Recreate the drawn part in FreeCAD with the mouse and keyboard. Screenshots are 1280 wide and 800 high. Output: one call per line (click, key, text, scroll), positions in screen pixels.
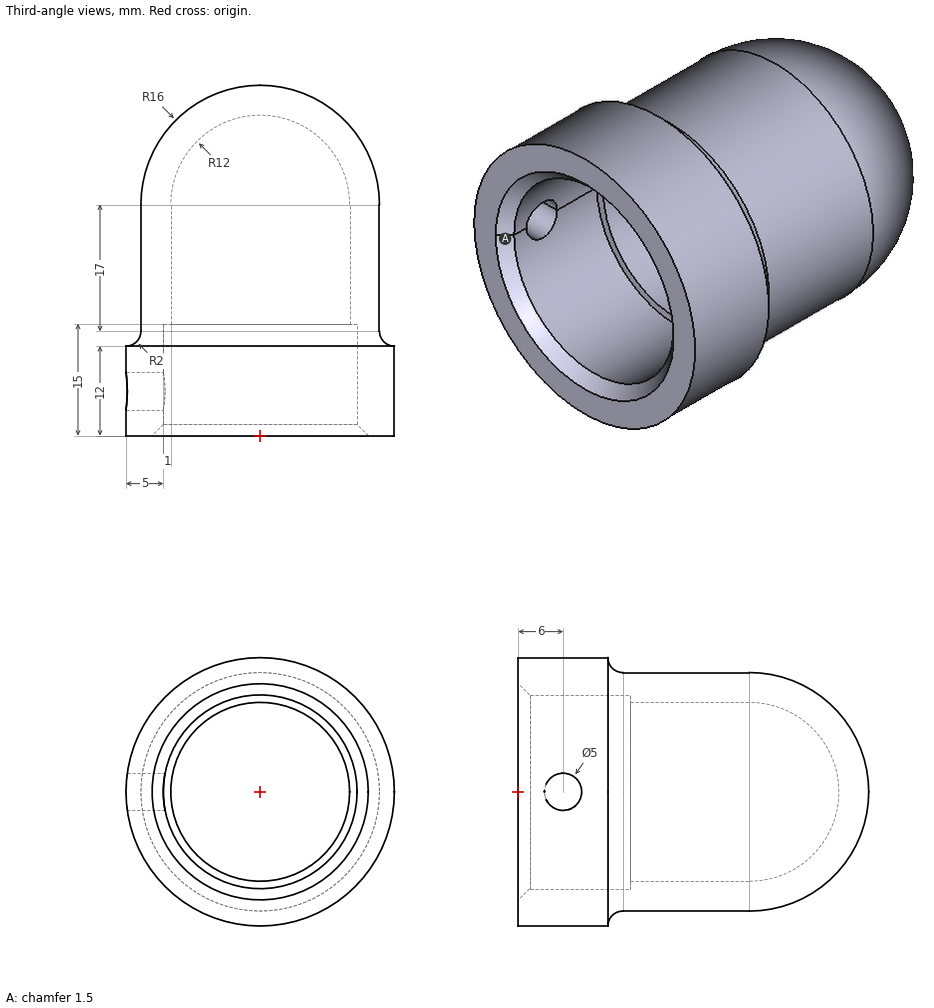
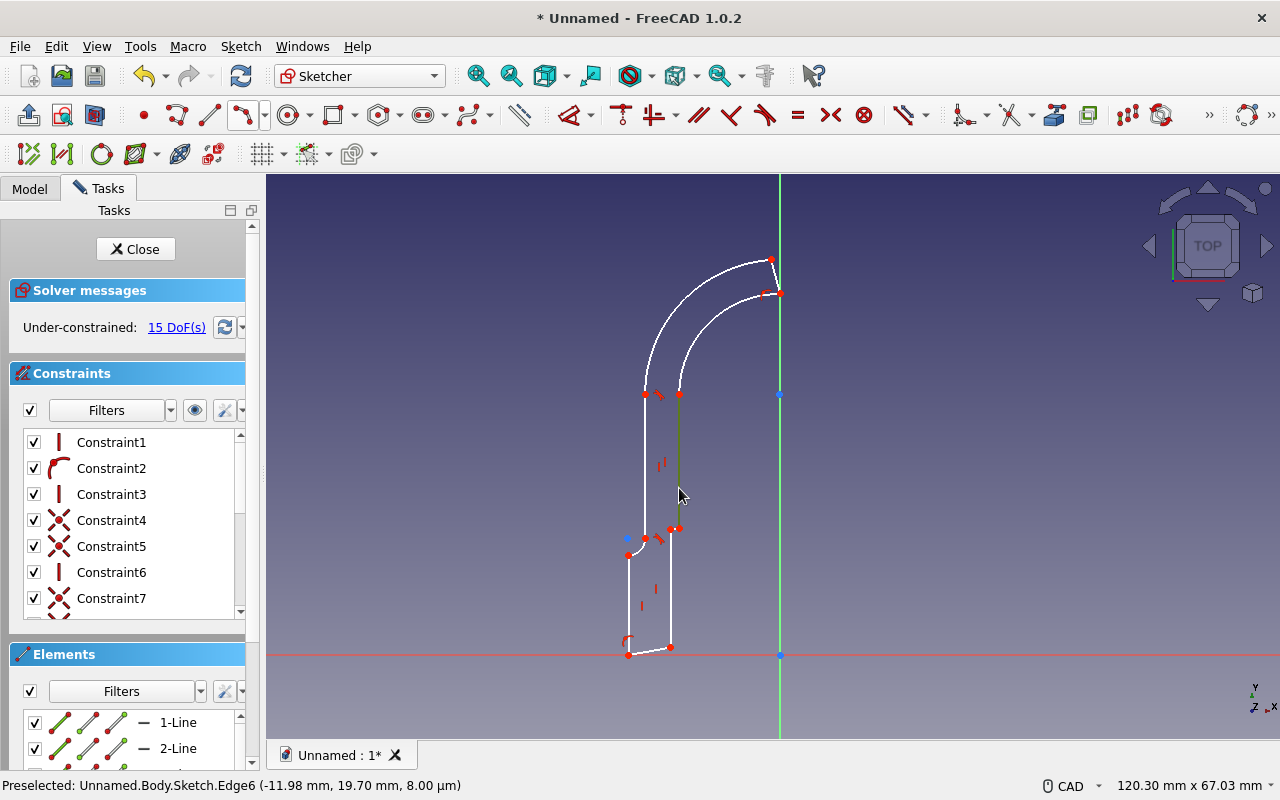
click(735, 305)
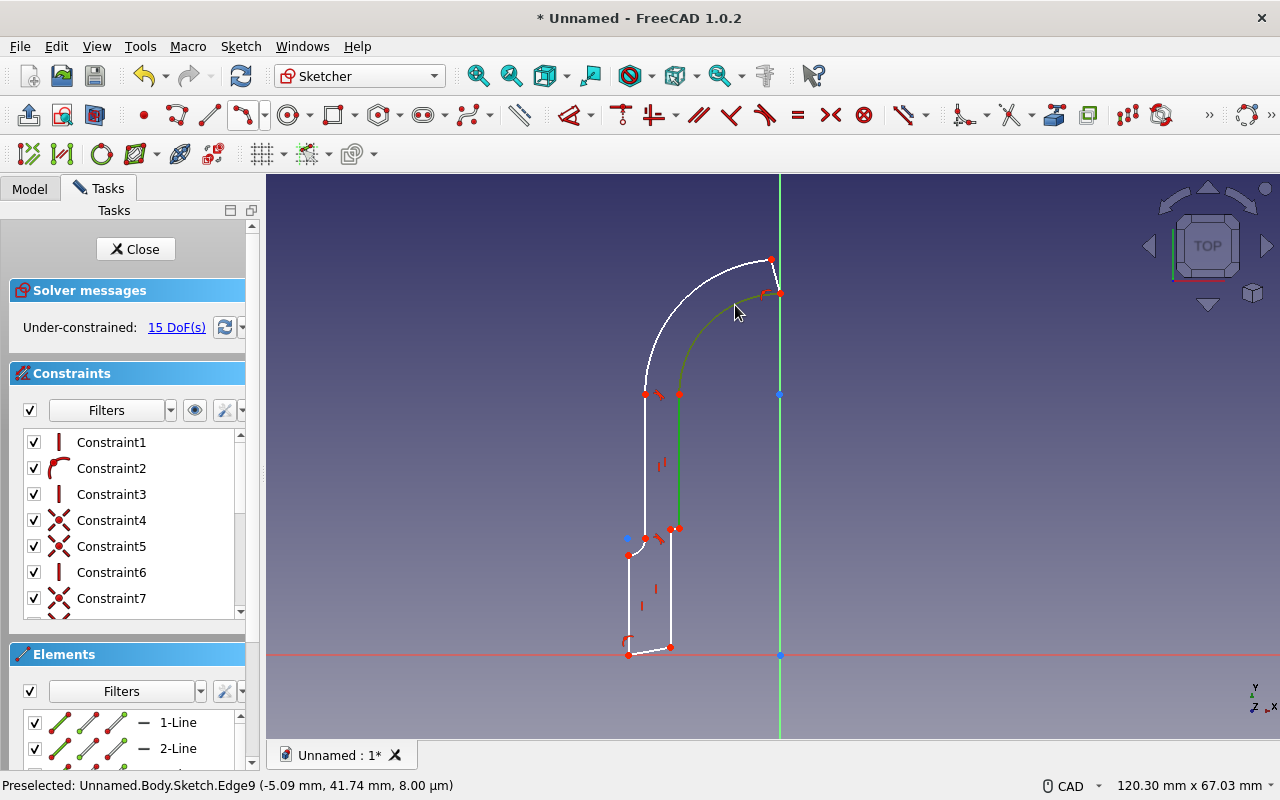
key(t)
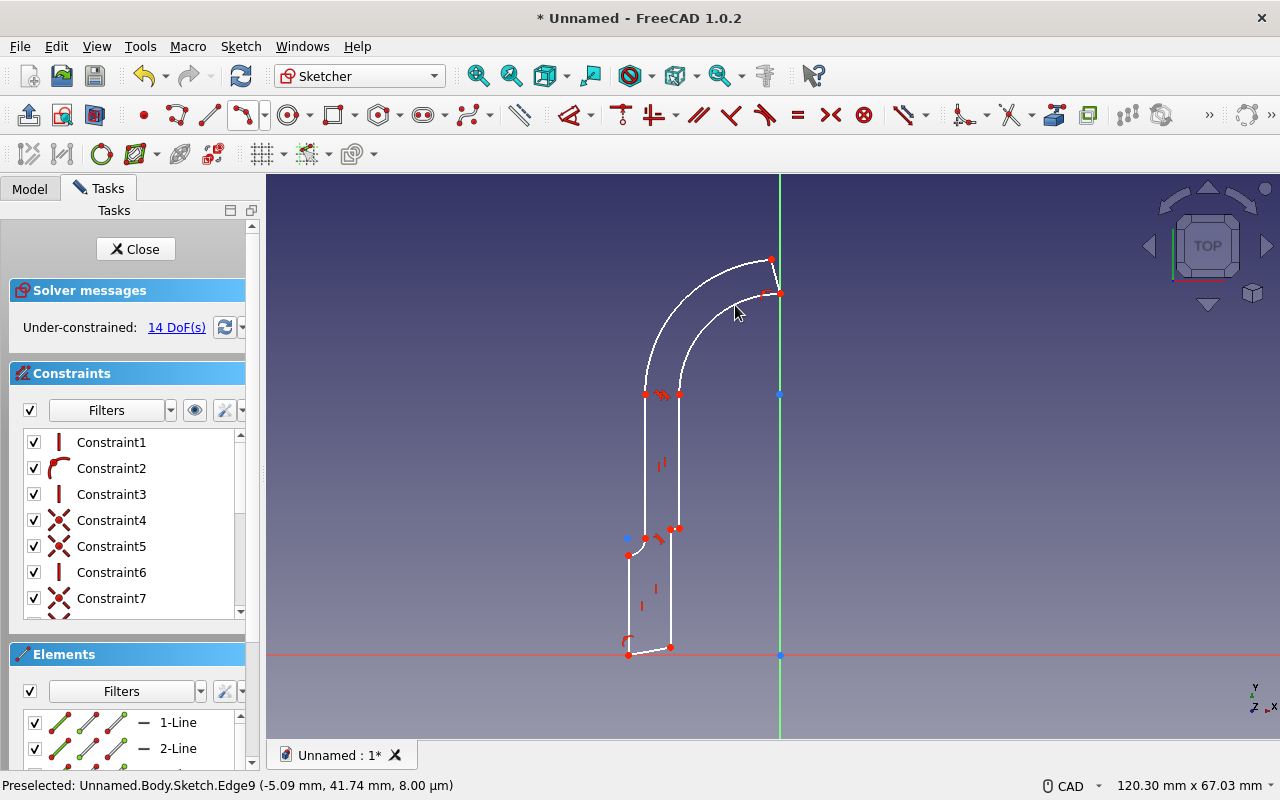
click(641, 653)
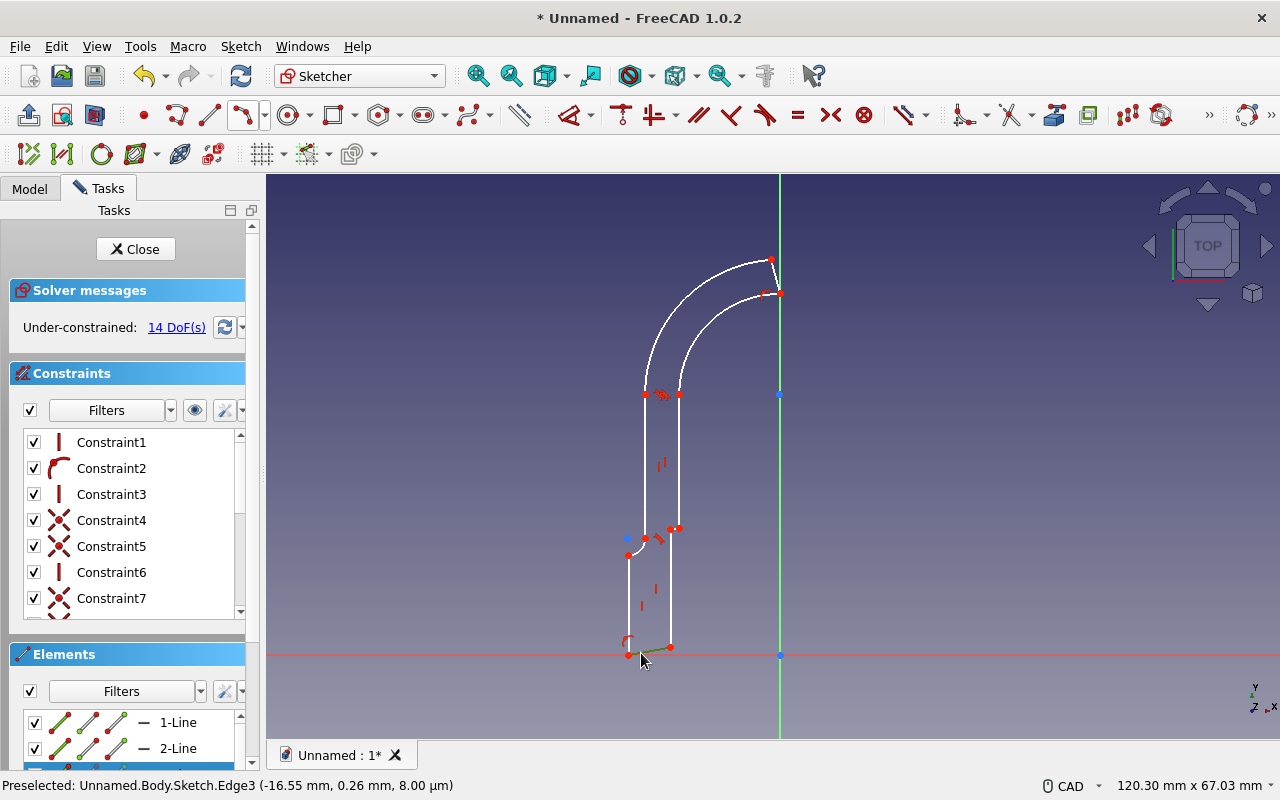
click(676, 116)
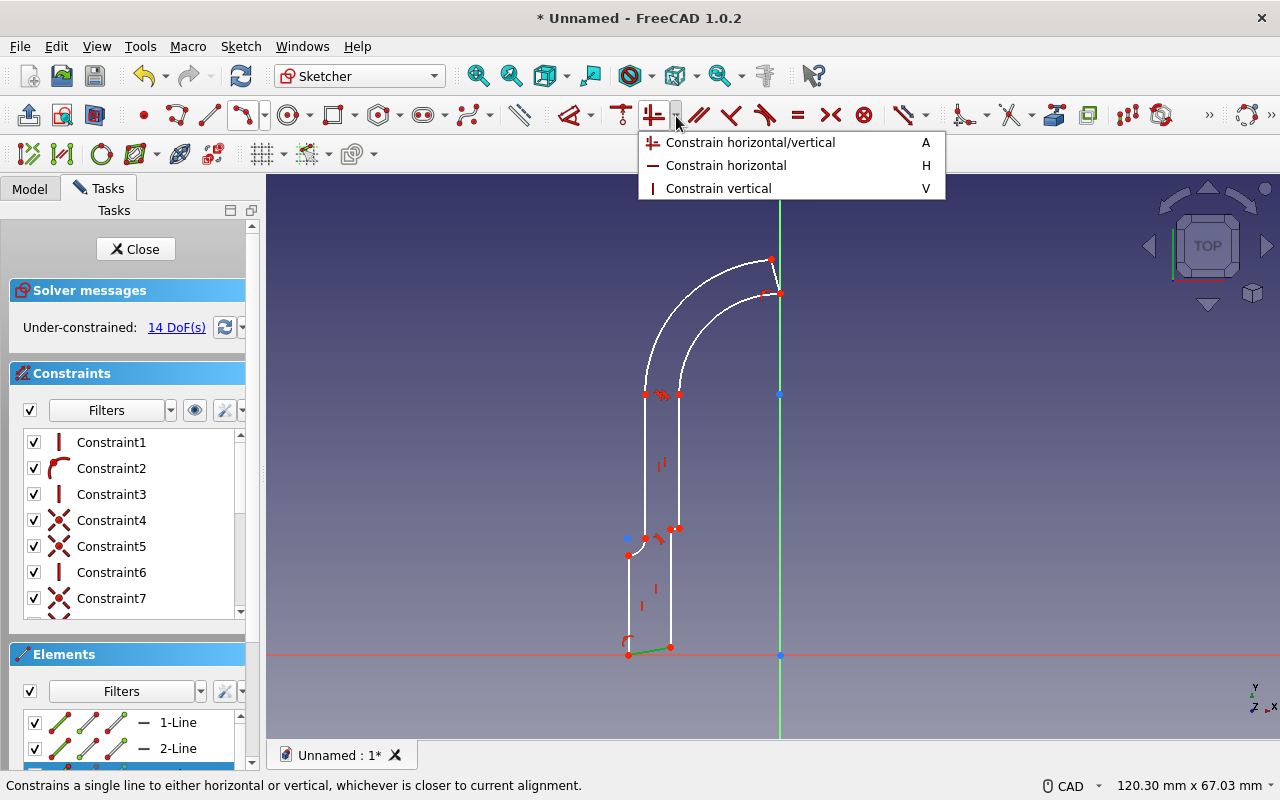
click(792, 166)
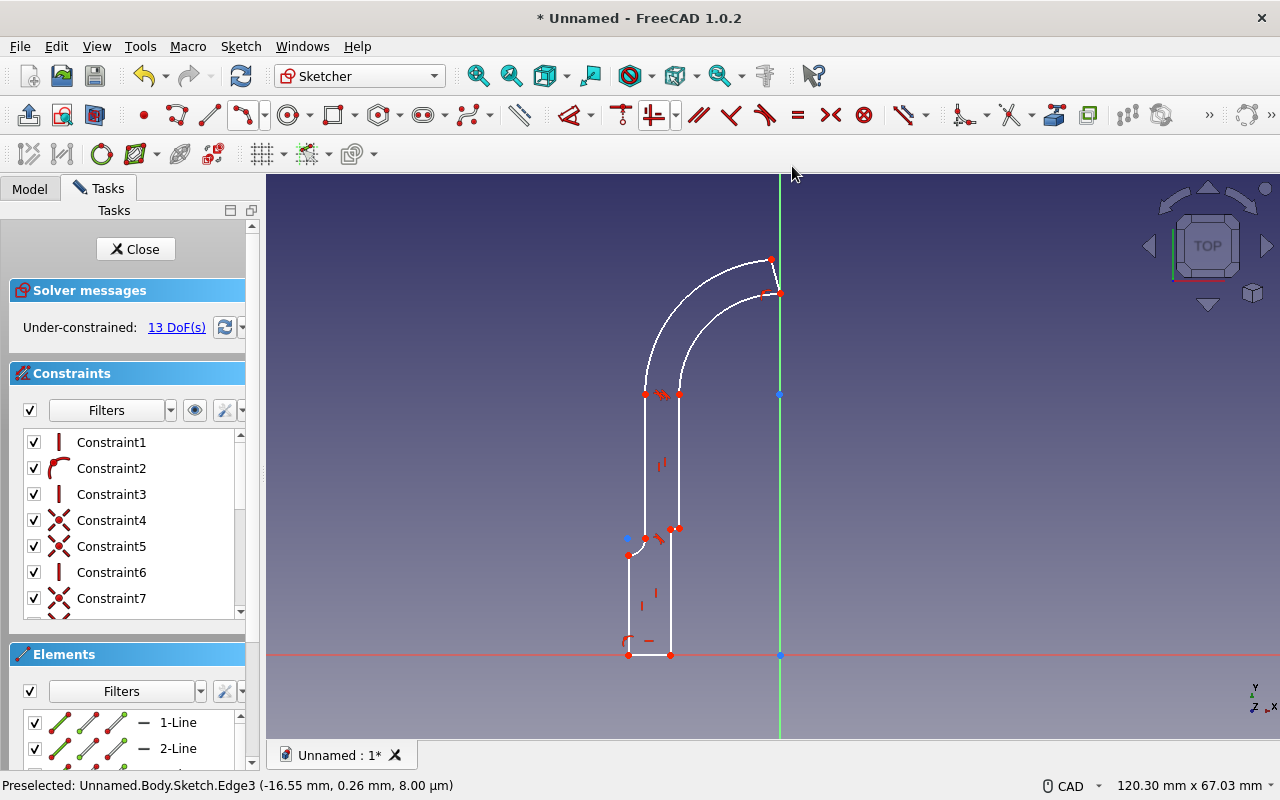
scroll(675, 529, up, 6)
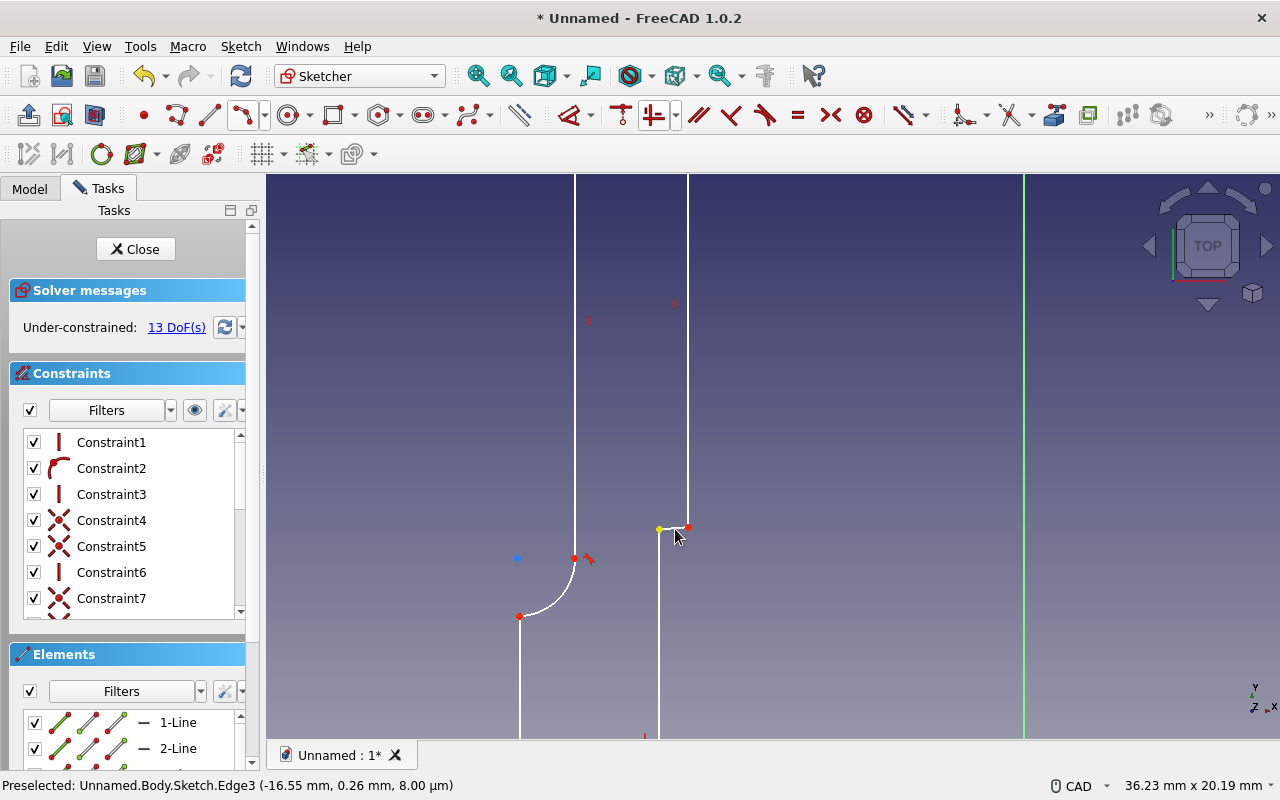
click(674, 528)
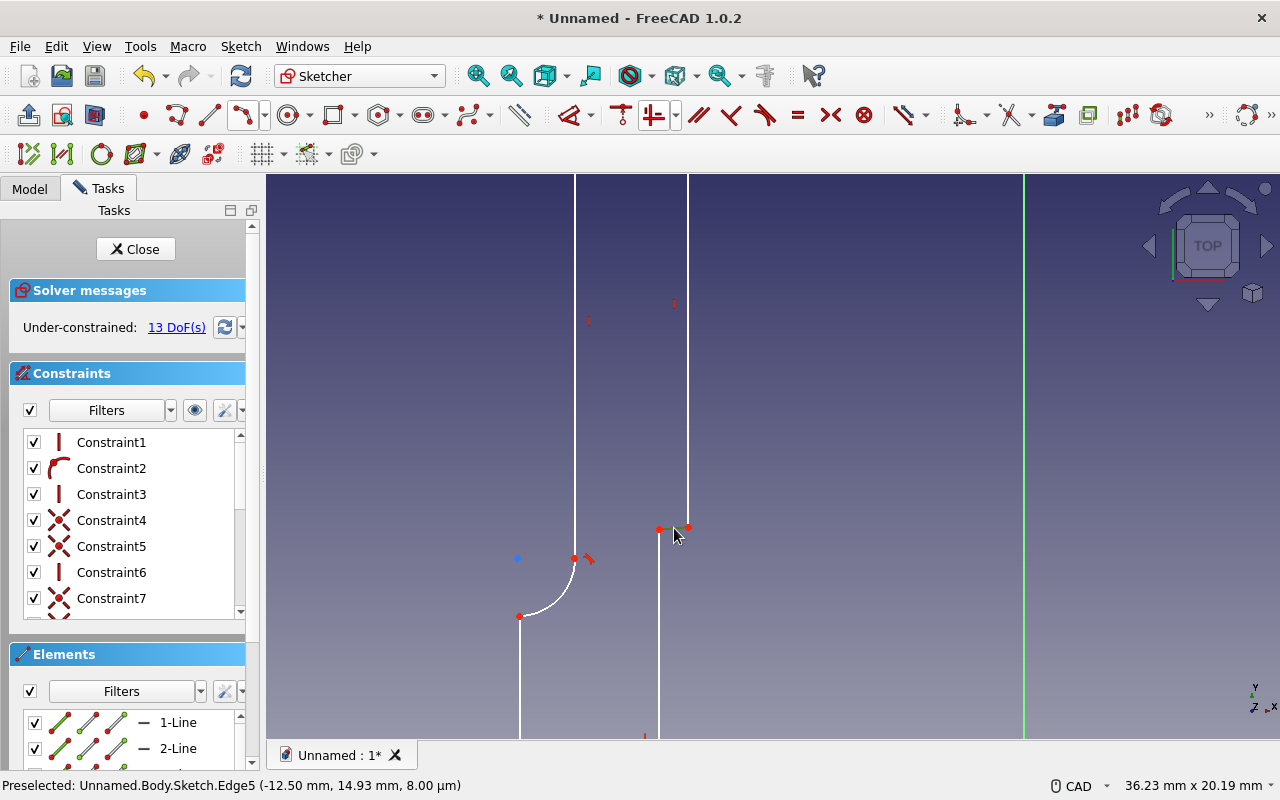
key(h)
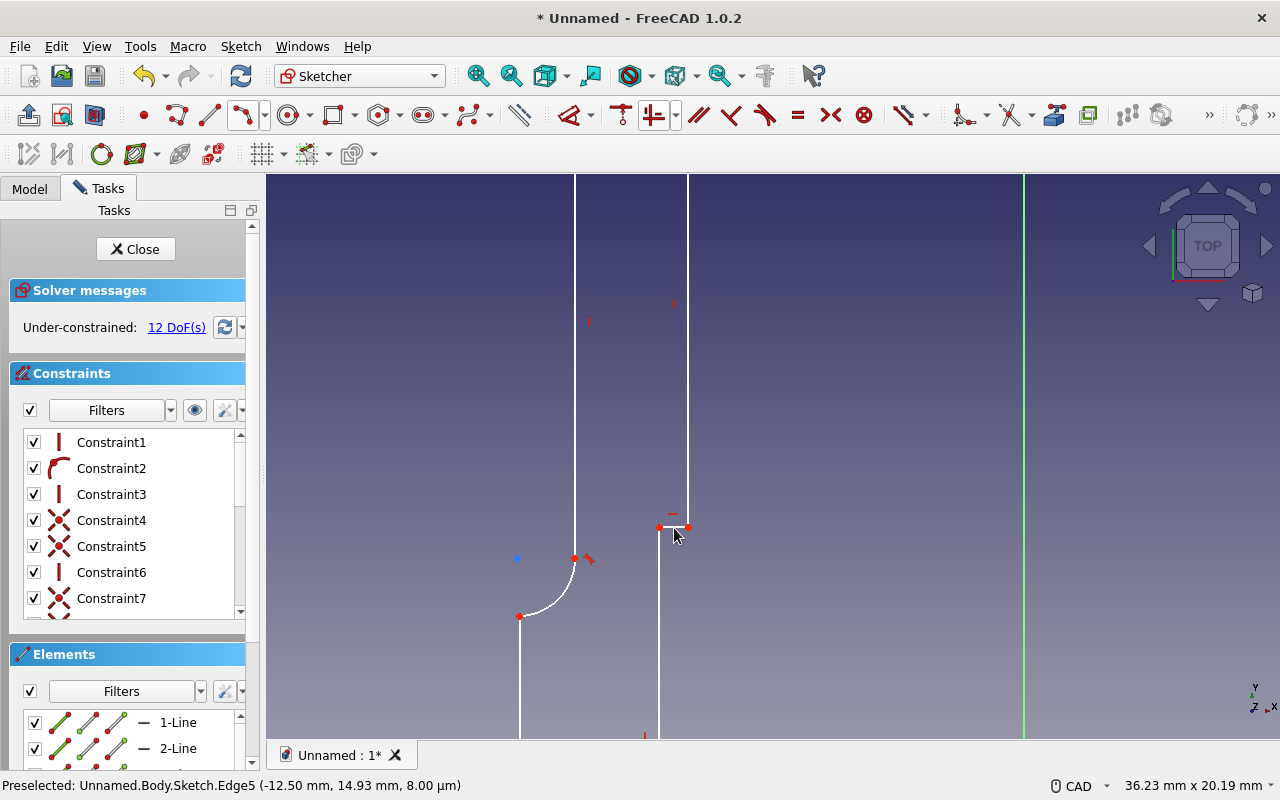
scroll(675, 529, down, 6)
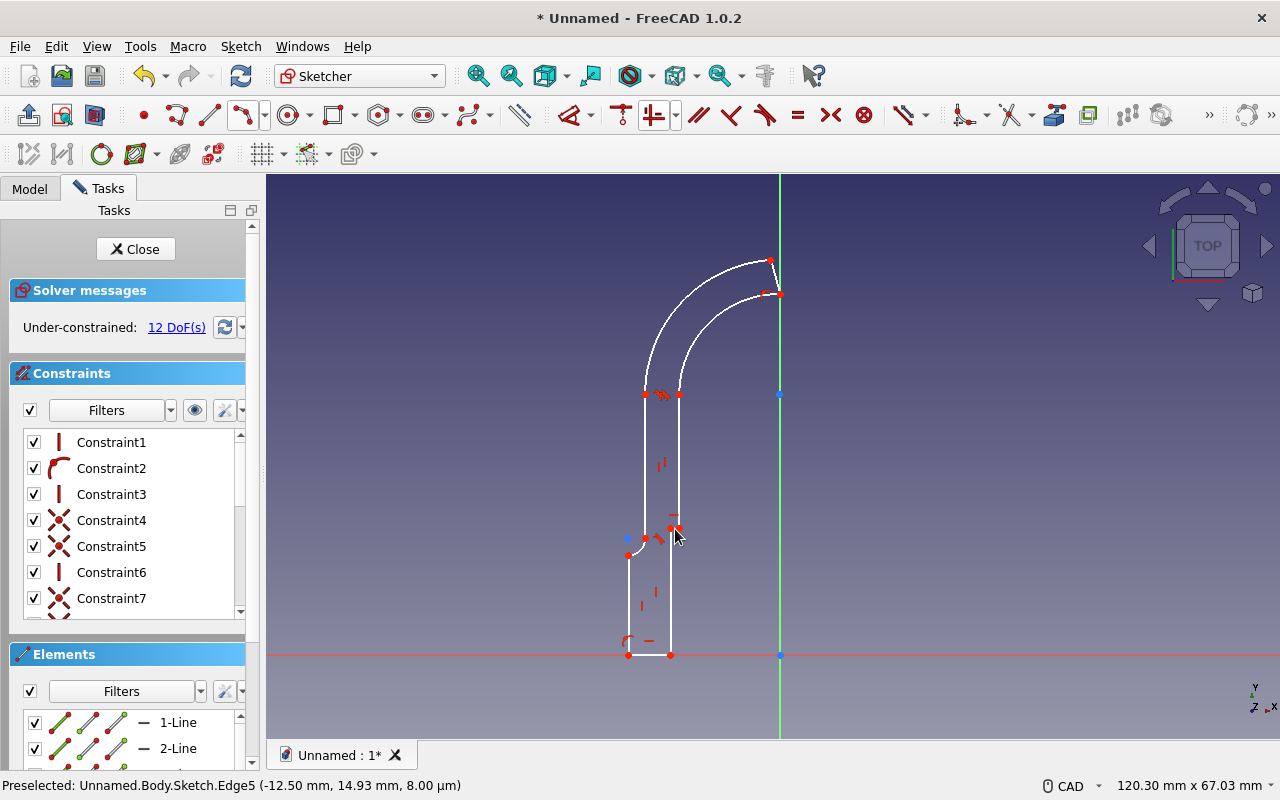
scroll(778, 284, up, 8)